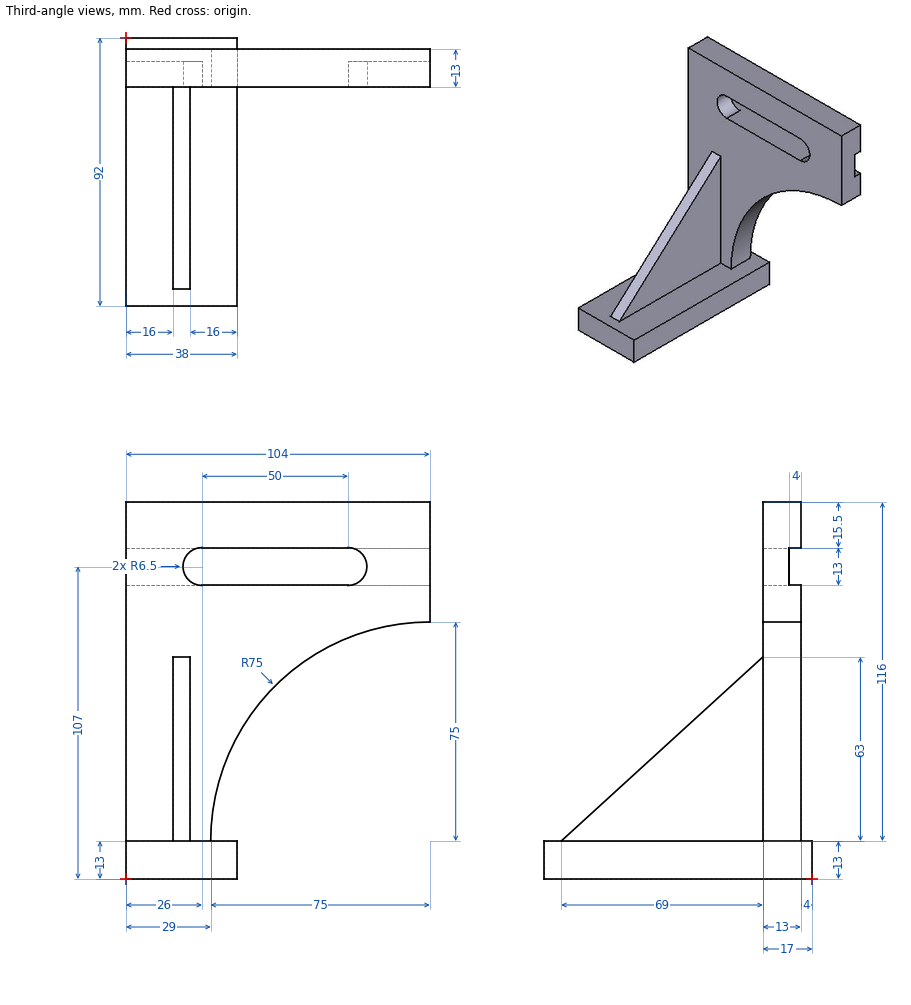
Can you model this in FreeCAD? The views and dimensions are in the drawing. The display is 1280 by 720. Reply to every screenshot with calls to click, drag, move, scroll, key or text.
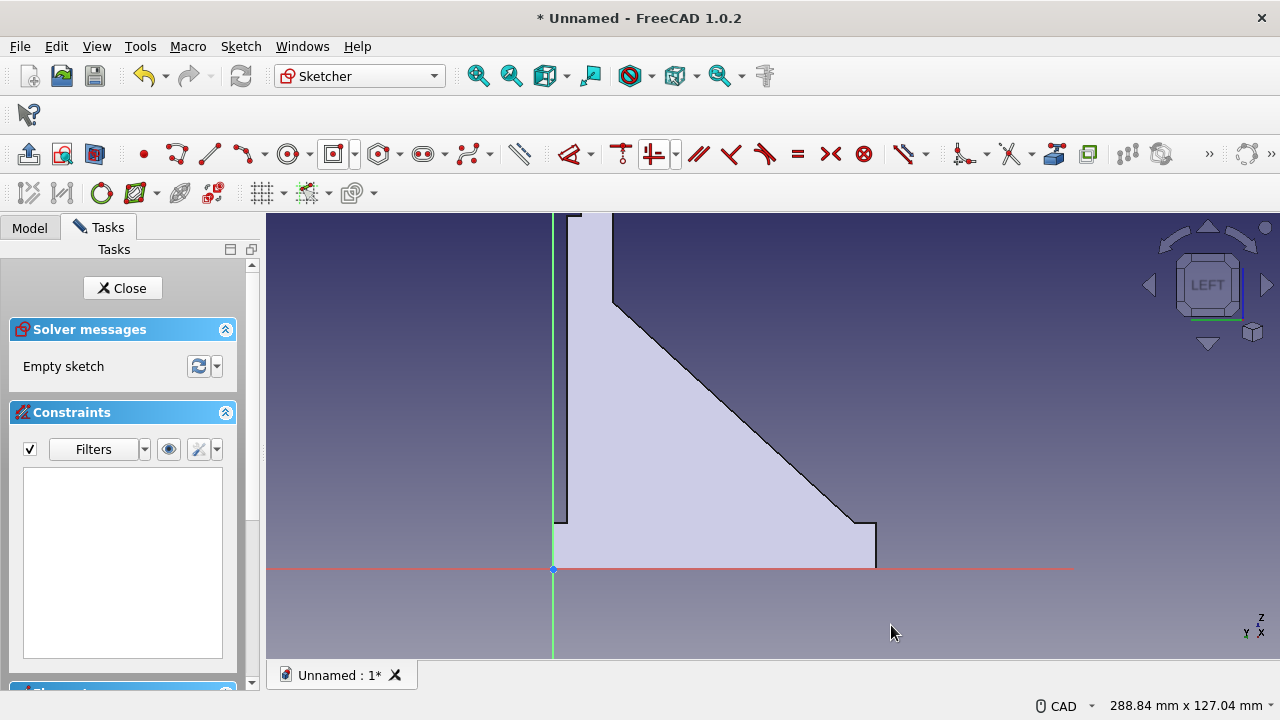
click(177, 154)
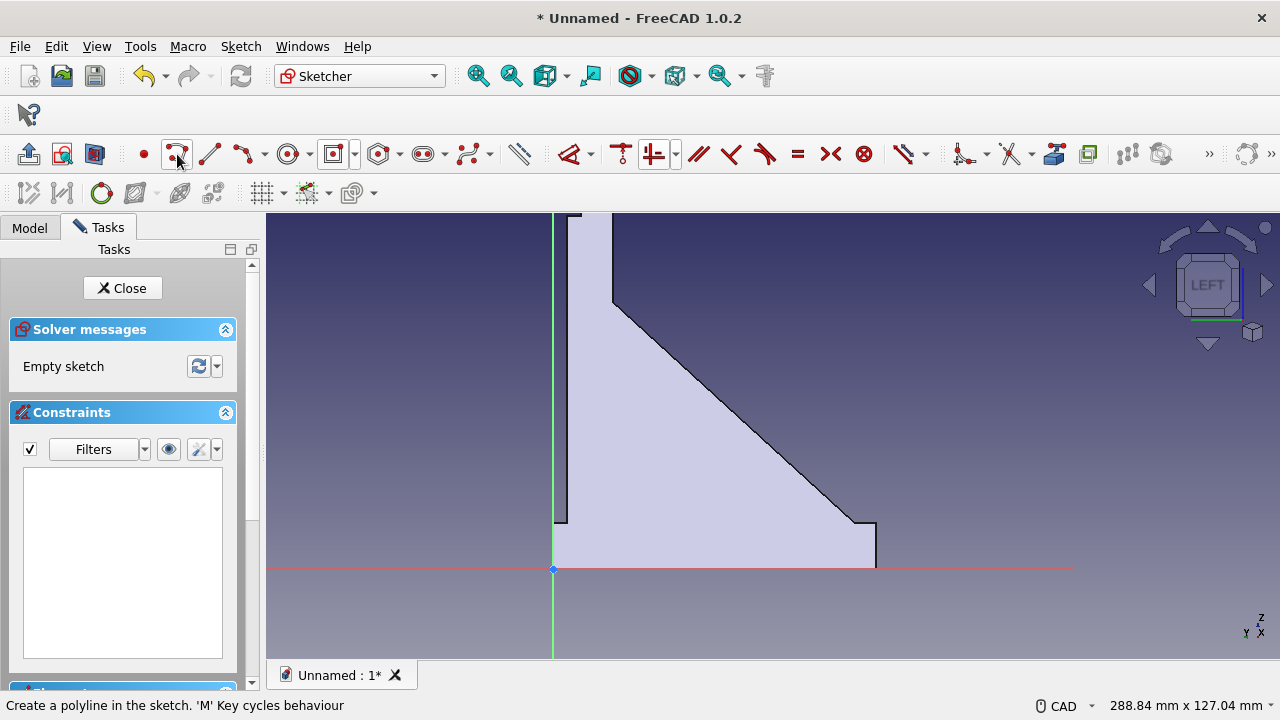
click(613, 523)
click(855, 523)
click(613, 302)
click(613, 524)
key(Escape)
key(Escape)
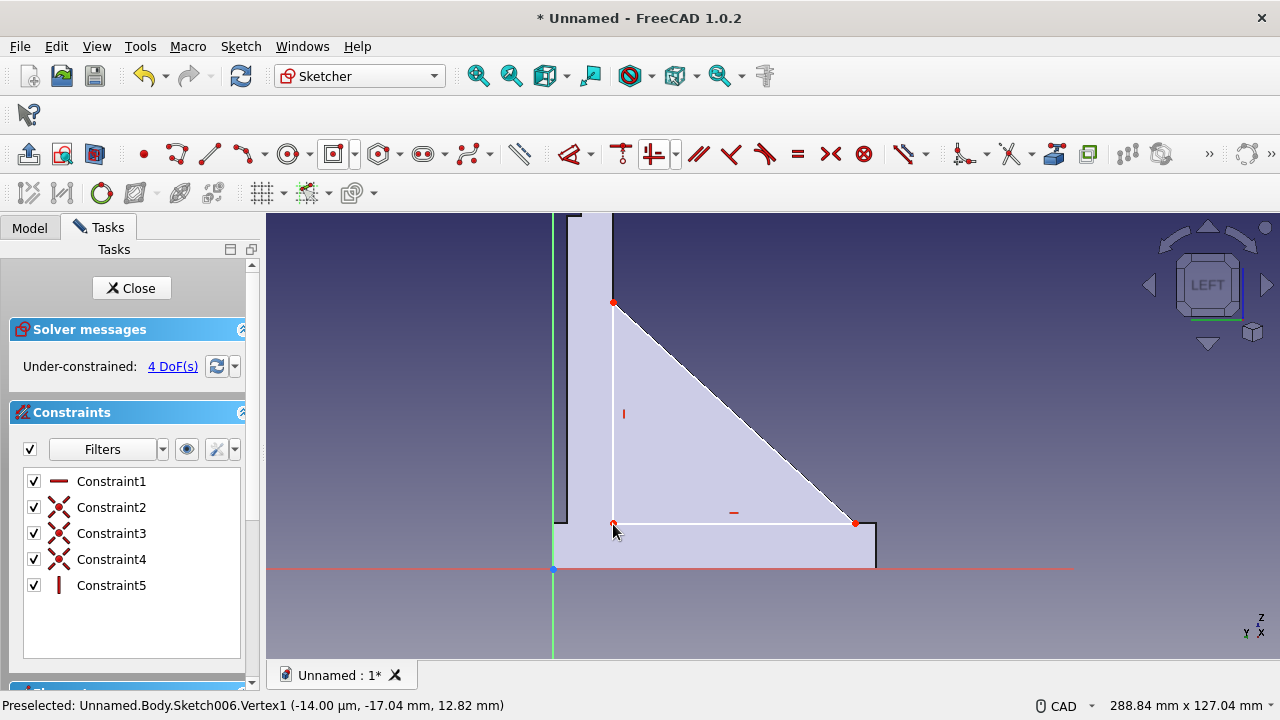
click(568, 154)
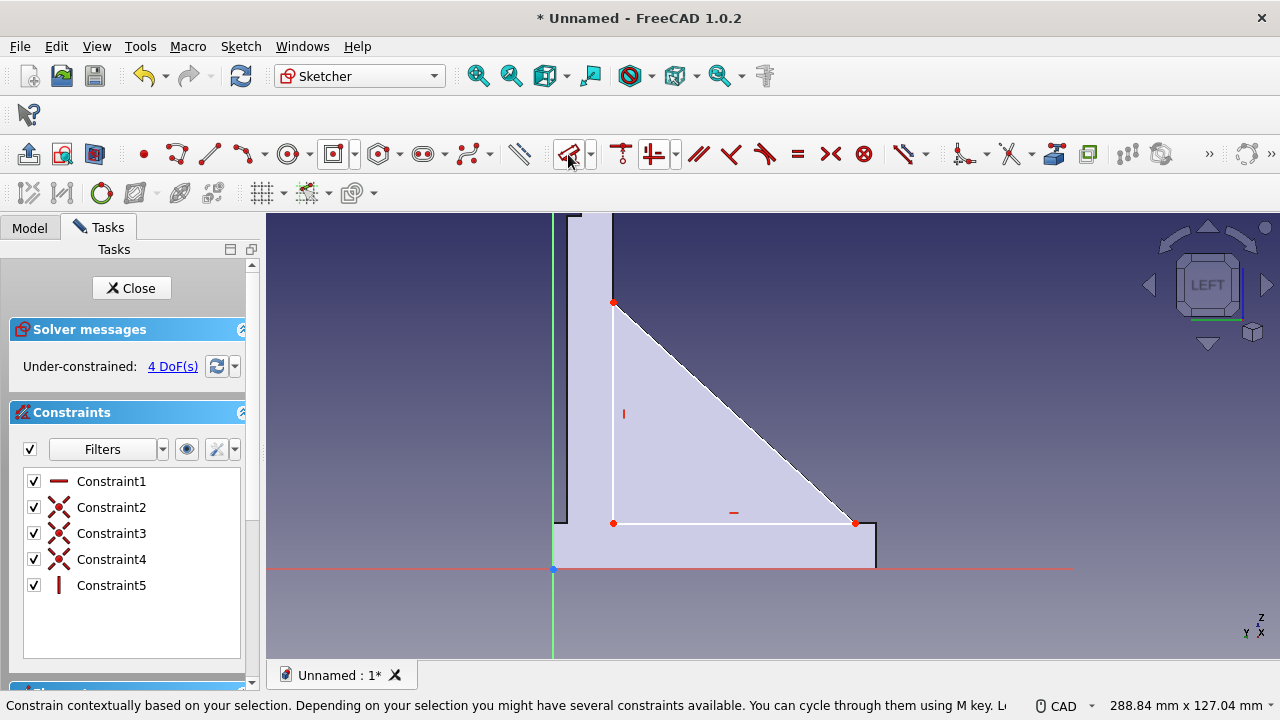
click(686, 524)
click(734, 490)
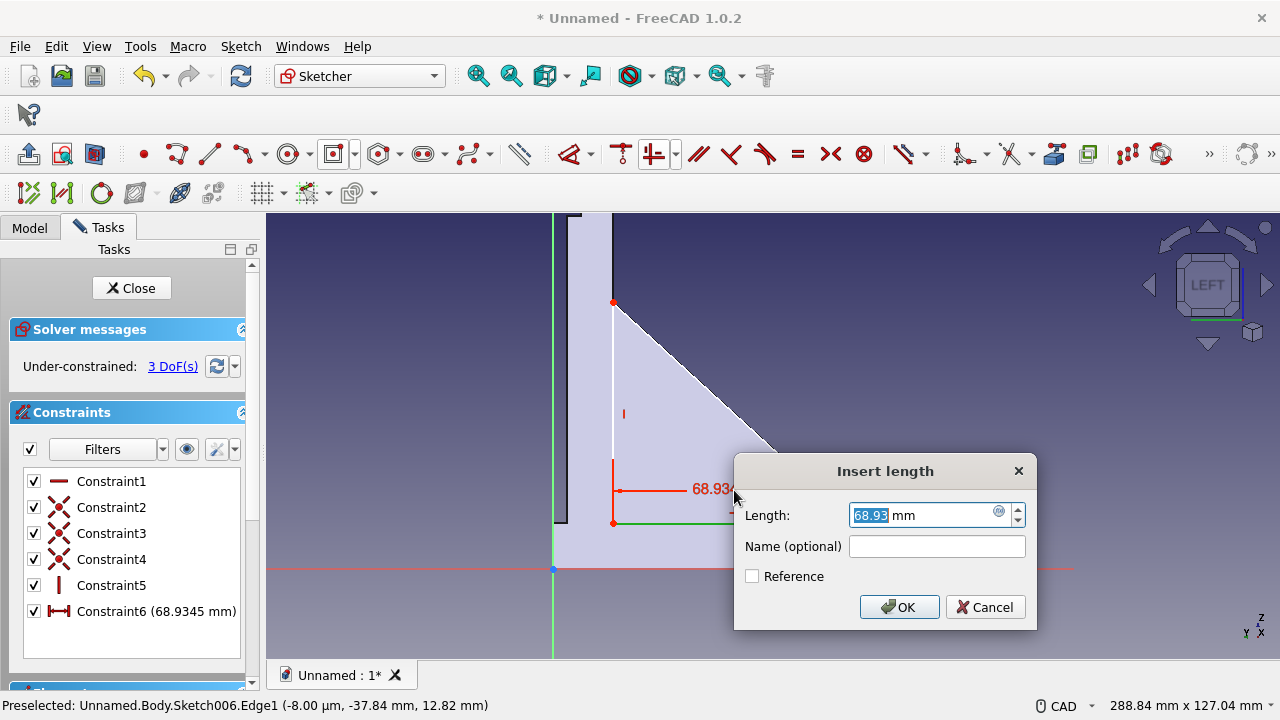
text(69)
key(Return)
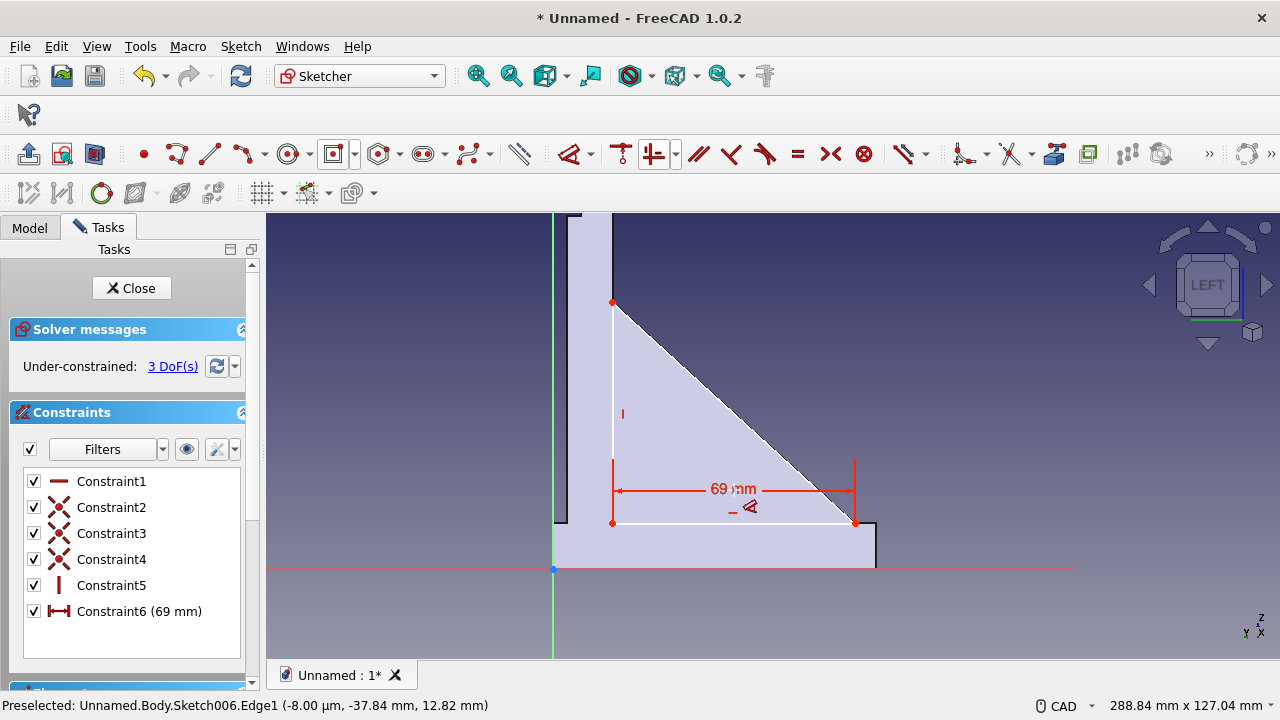
click(613, 369)
click(579, 414)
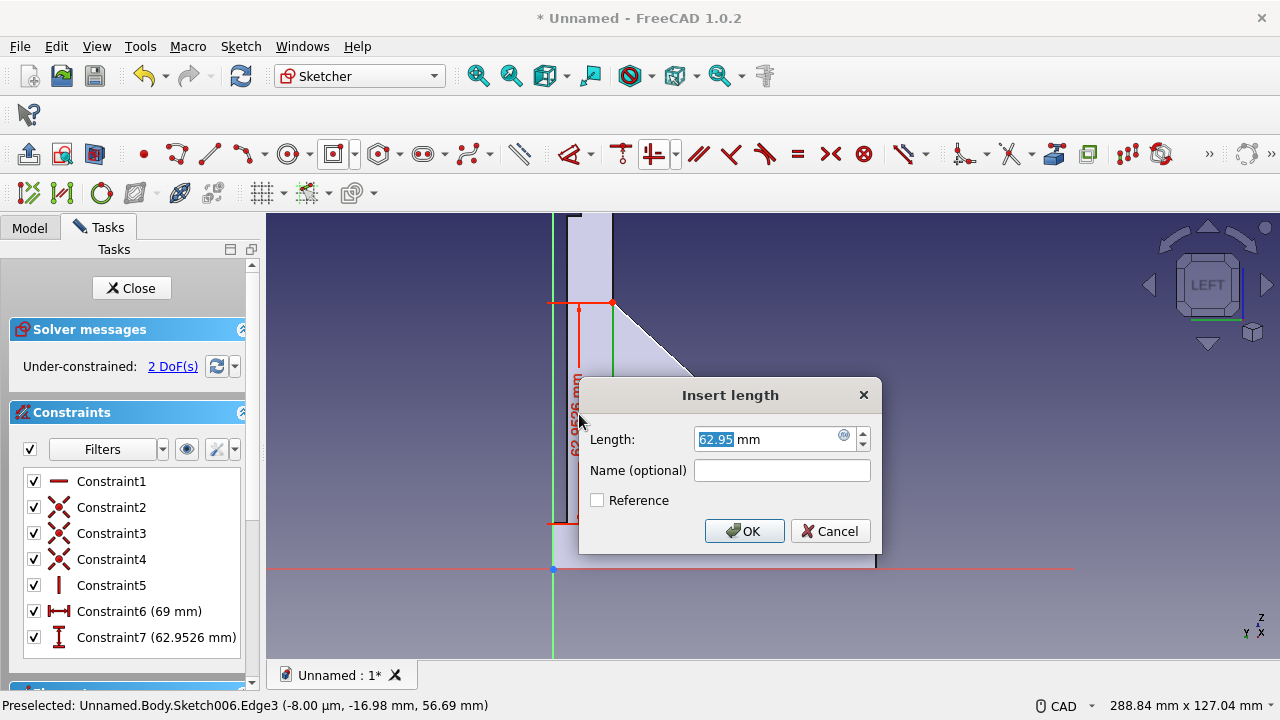
text(63)
key(Return)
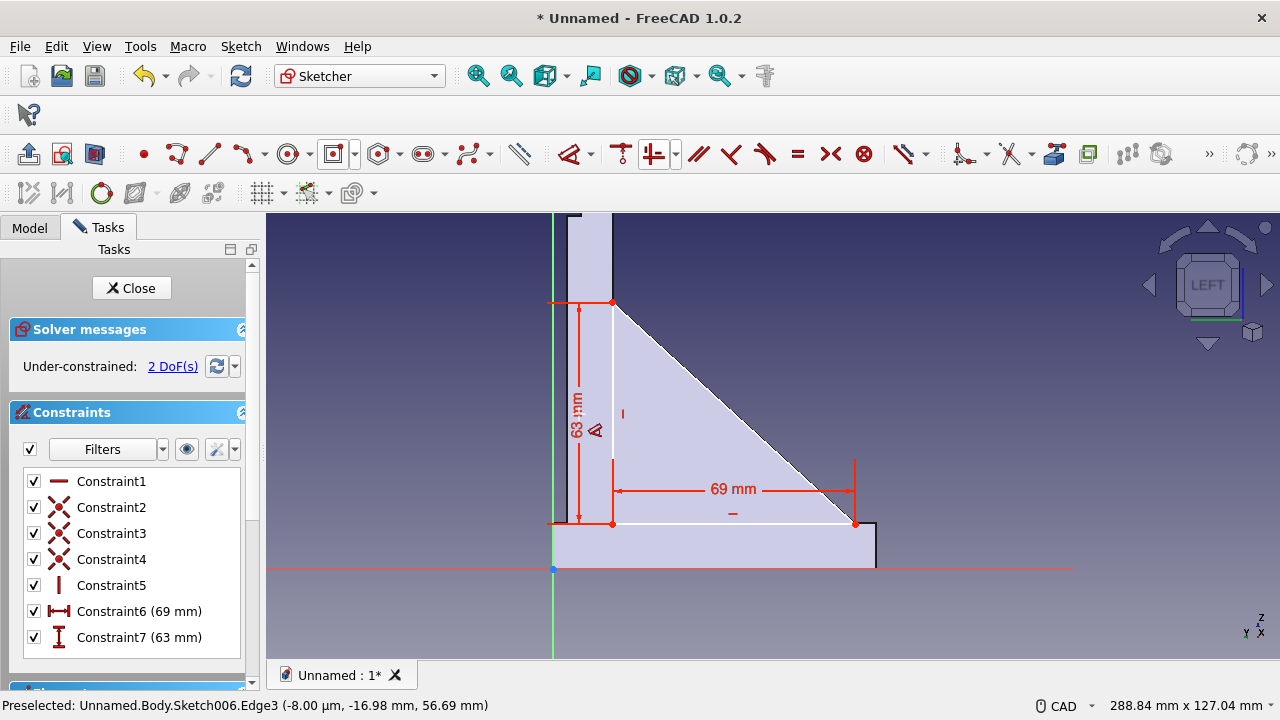
click(613, 524)
click(583, 603)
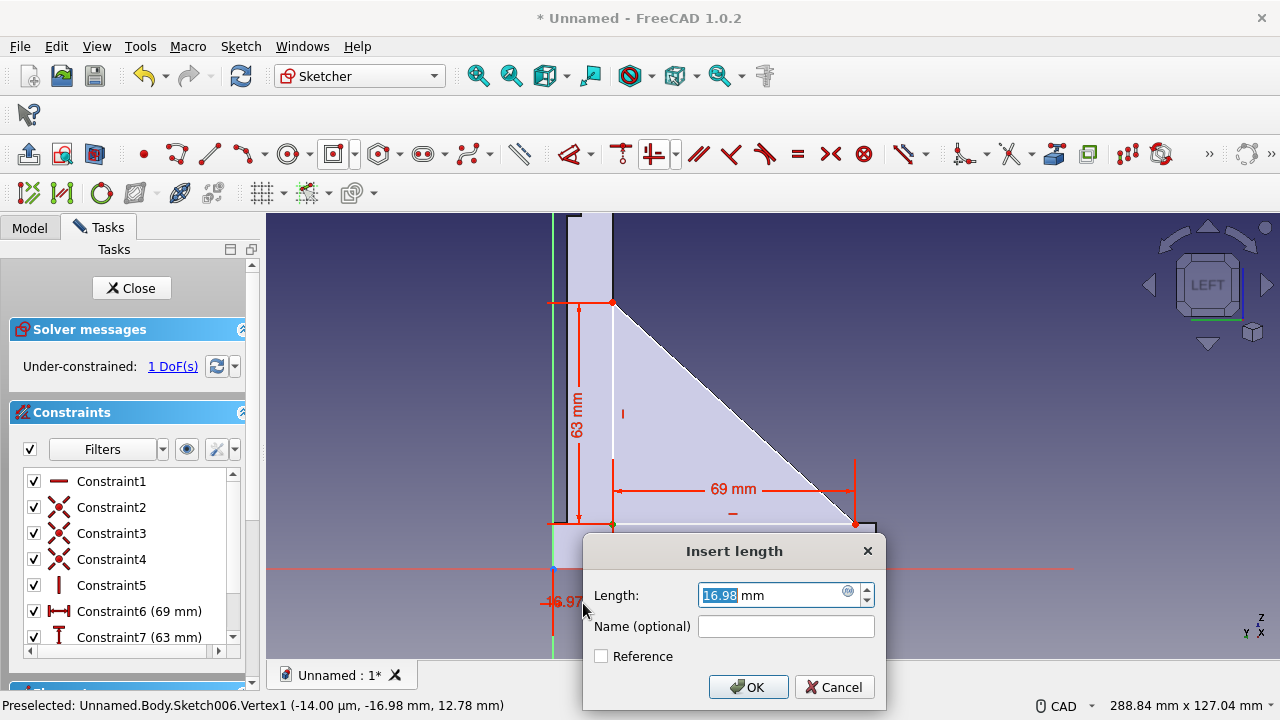
text(17)
key(Return)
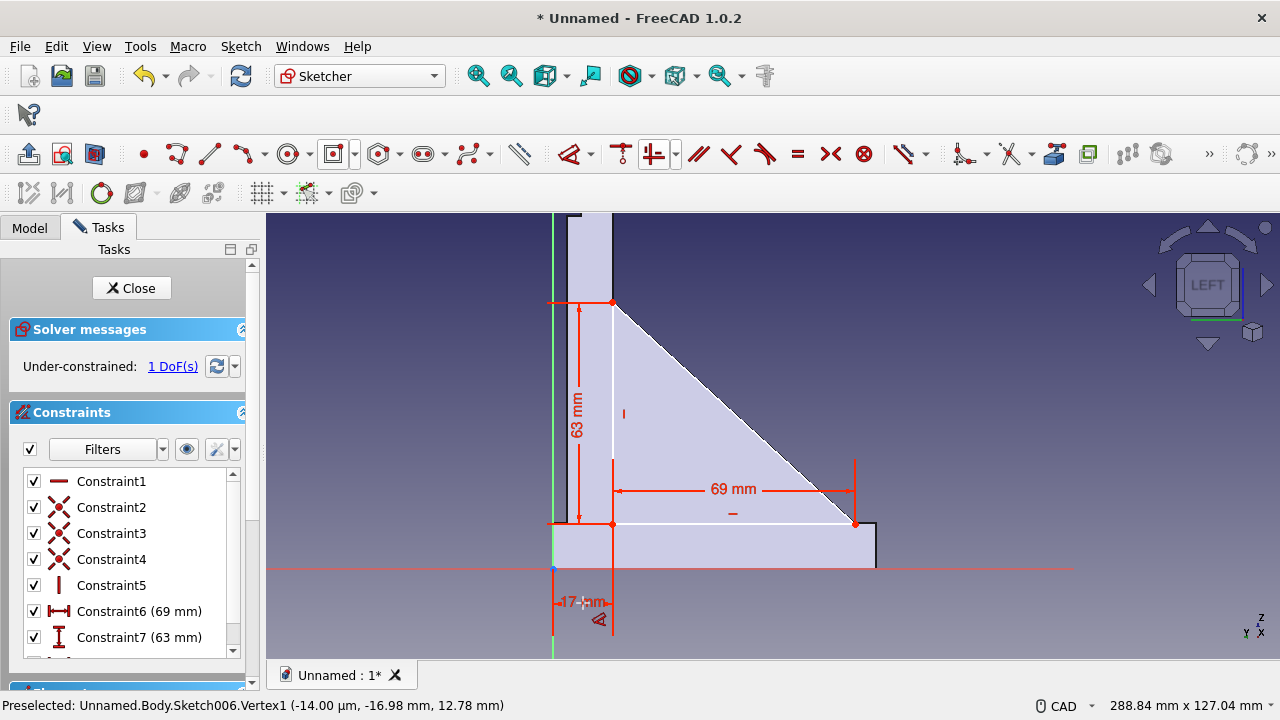
click(613, 524)
click(519, 547)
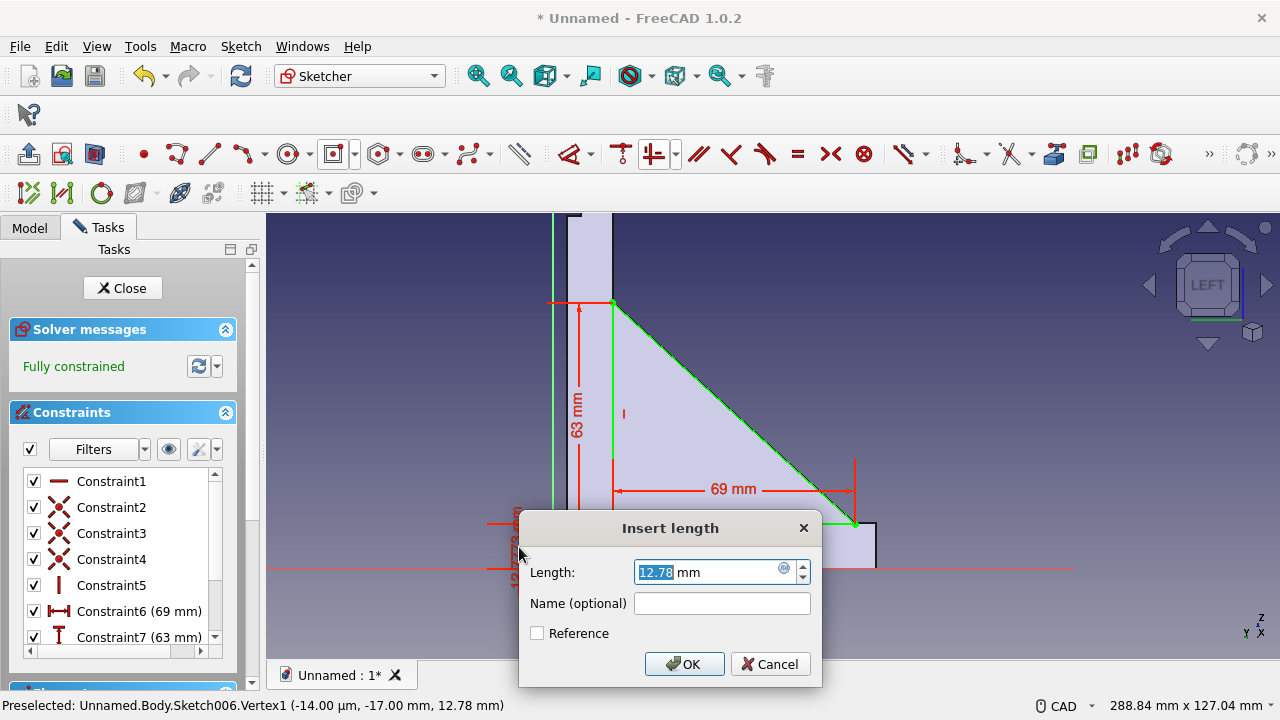
text(13)
key(Return)
key(Escape)